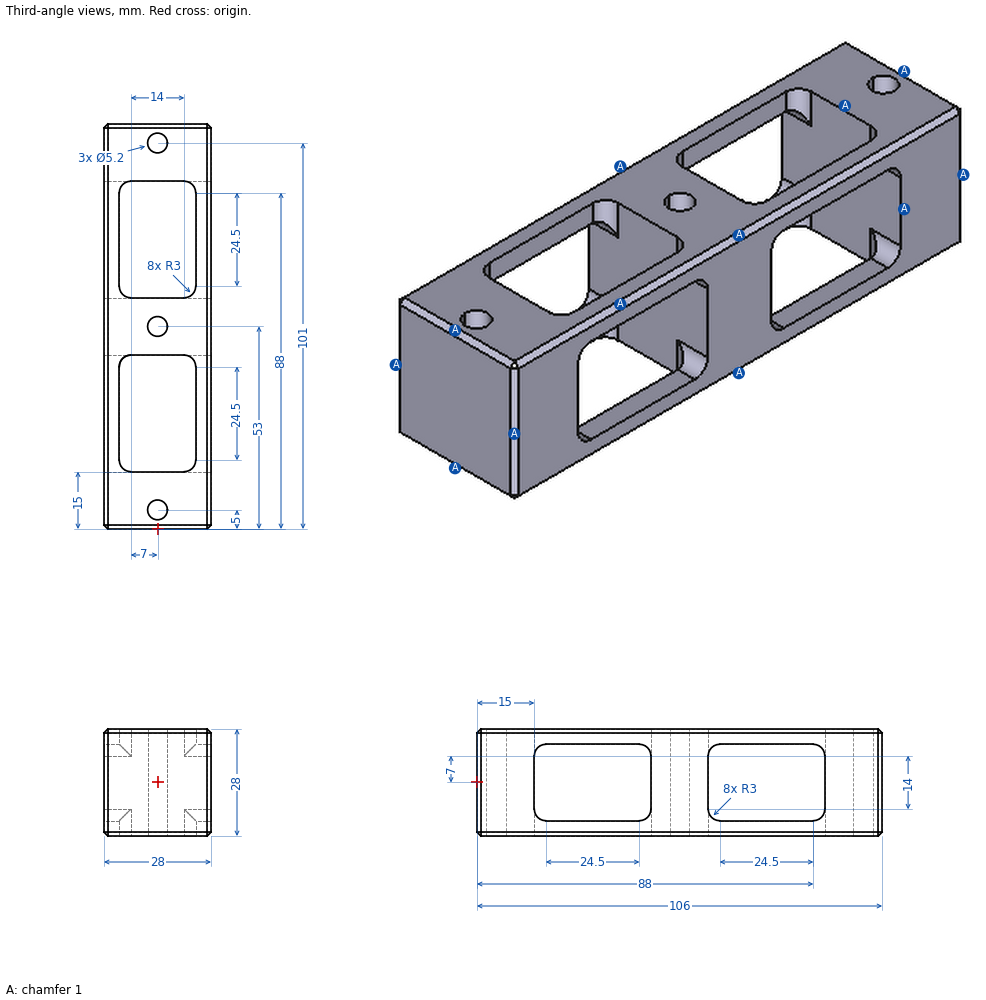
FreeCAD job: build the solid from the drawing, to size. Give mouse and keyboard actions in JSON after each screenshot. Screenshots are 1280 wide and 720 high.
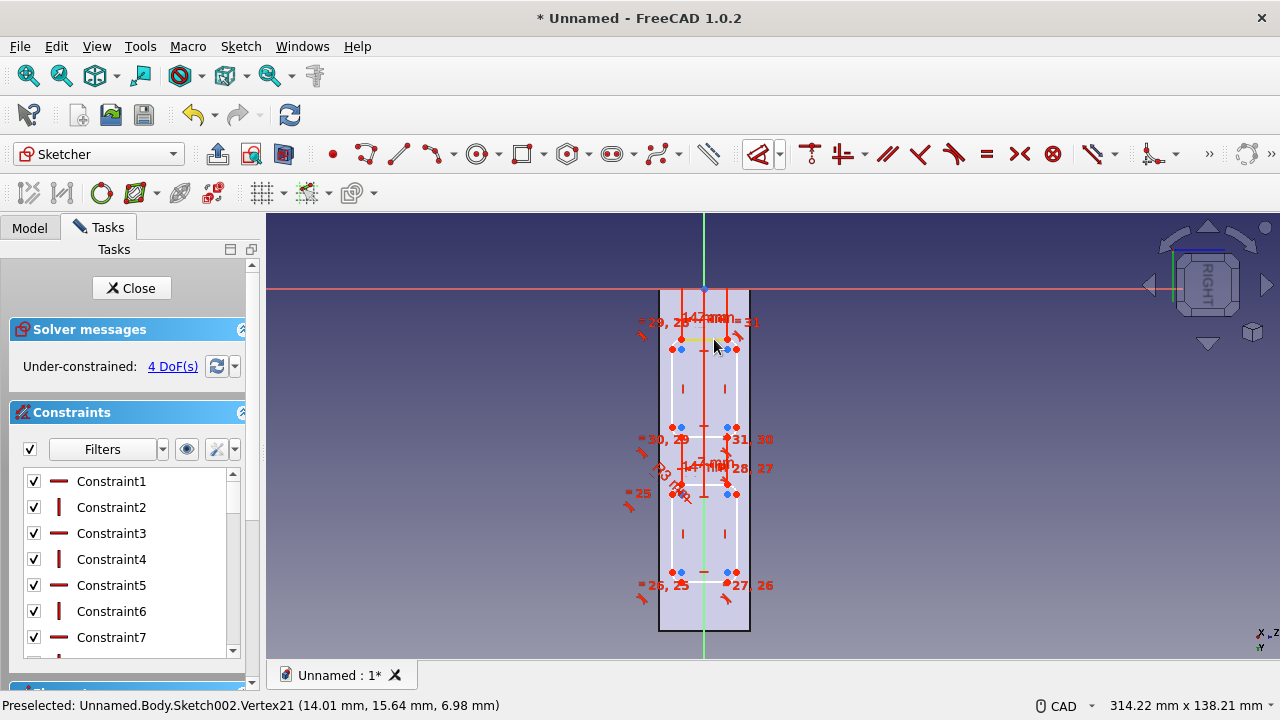
{"action": "scroll", "coordinate": [672, 573], "scroll_direction": "up", "scroll_amount": 2}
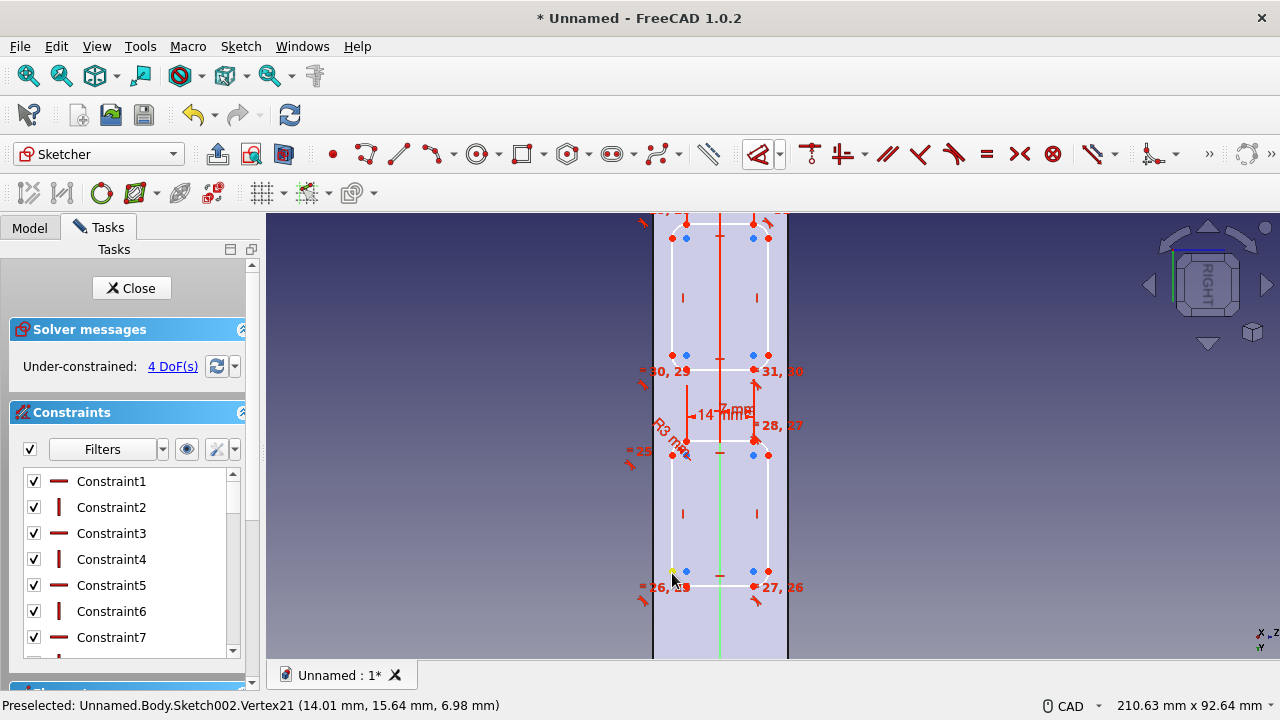
{"action": "left_click", "coordinate": [672, 572]}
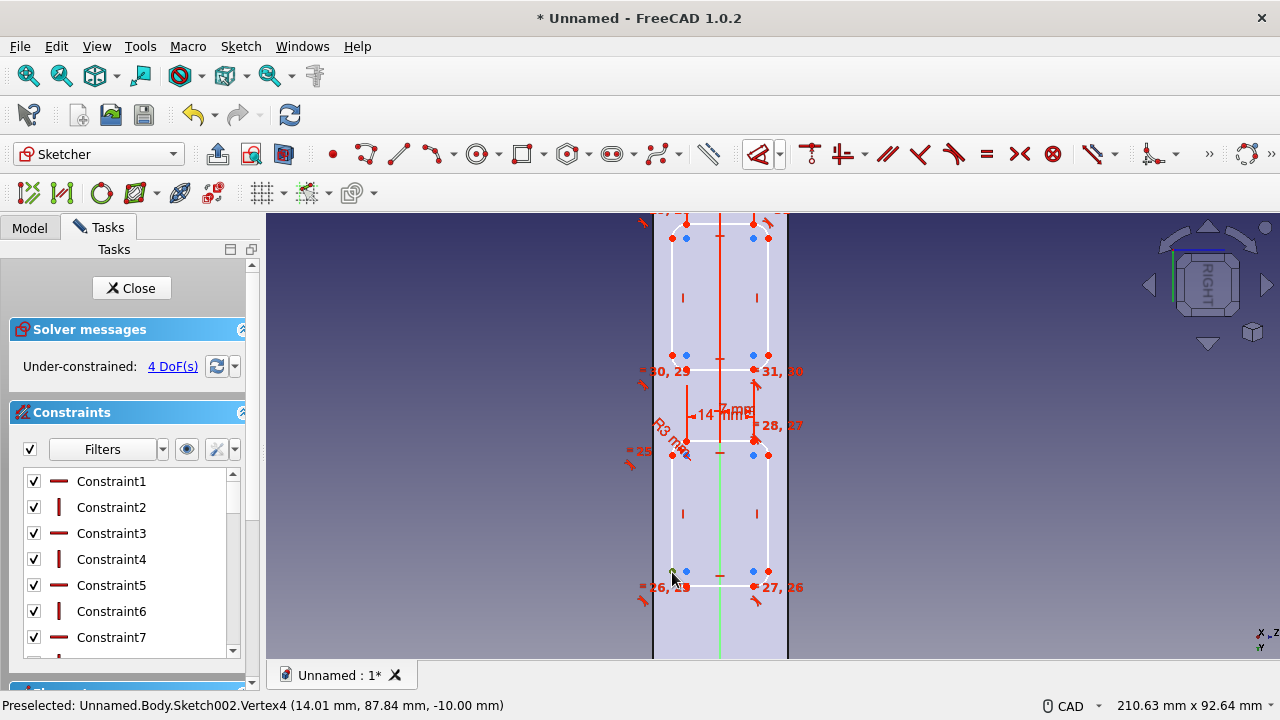
{"action": "key", "text": "i"}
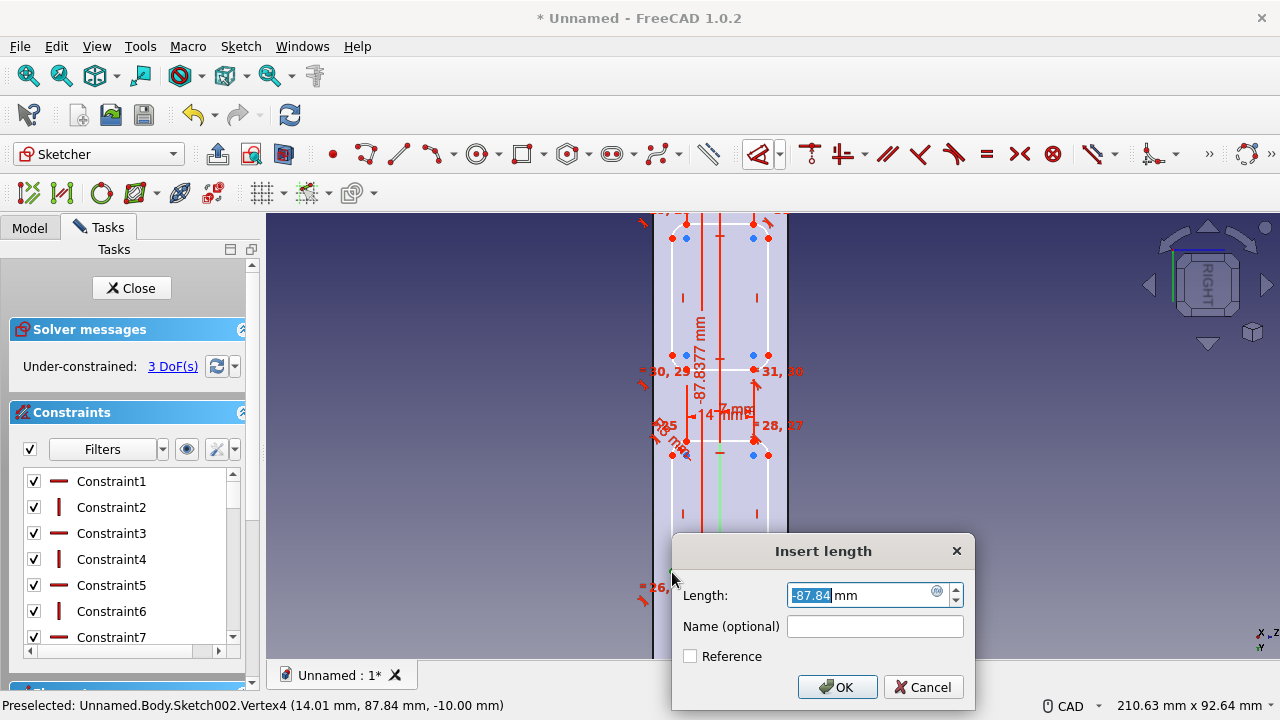
{"action": "type", "text": "-88"}
{"action": "key", "text": "Return"}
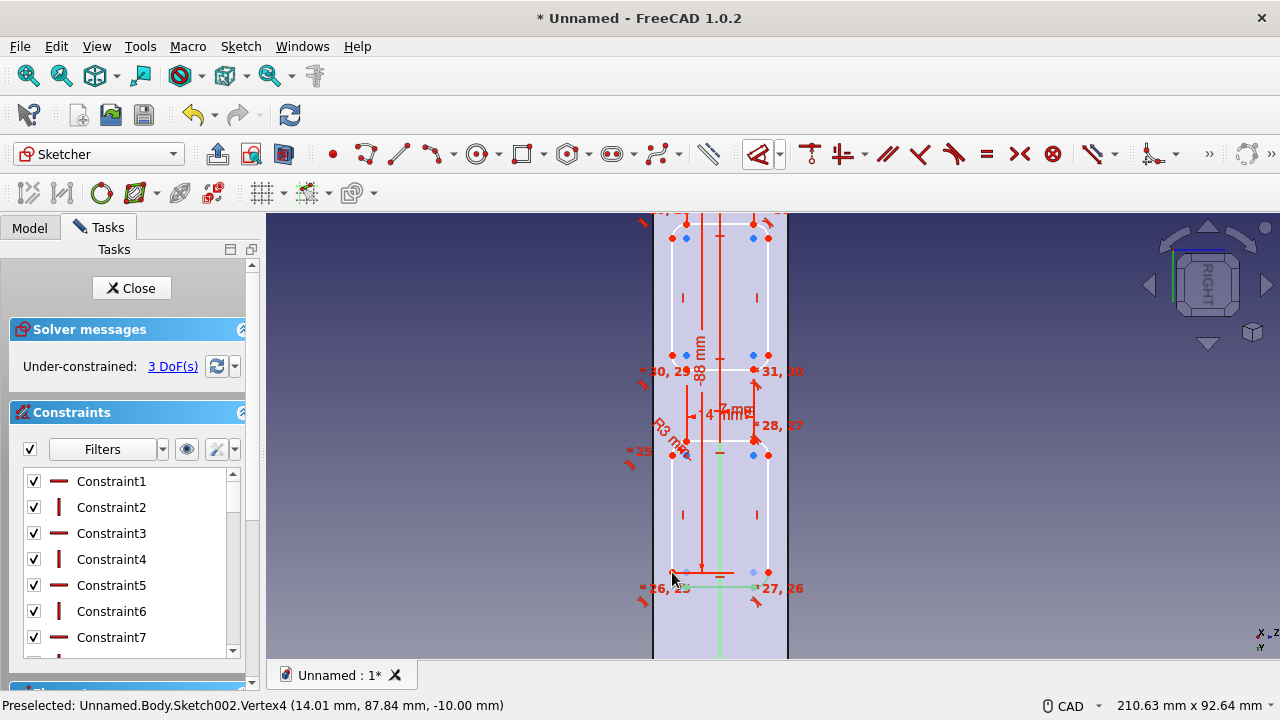
{"action": "scroll", "coordinate": [672, 574], "scroll_direction": "down", "scroll_amount": 2}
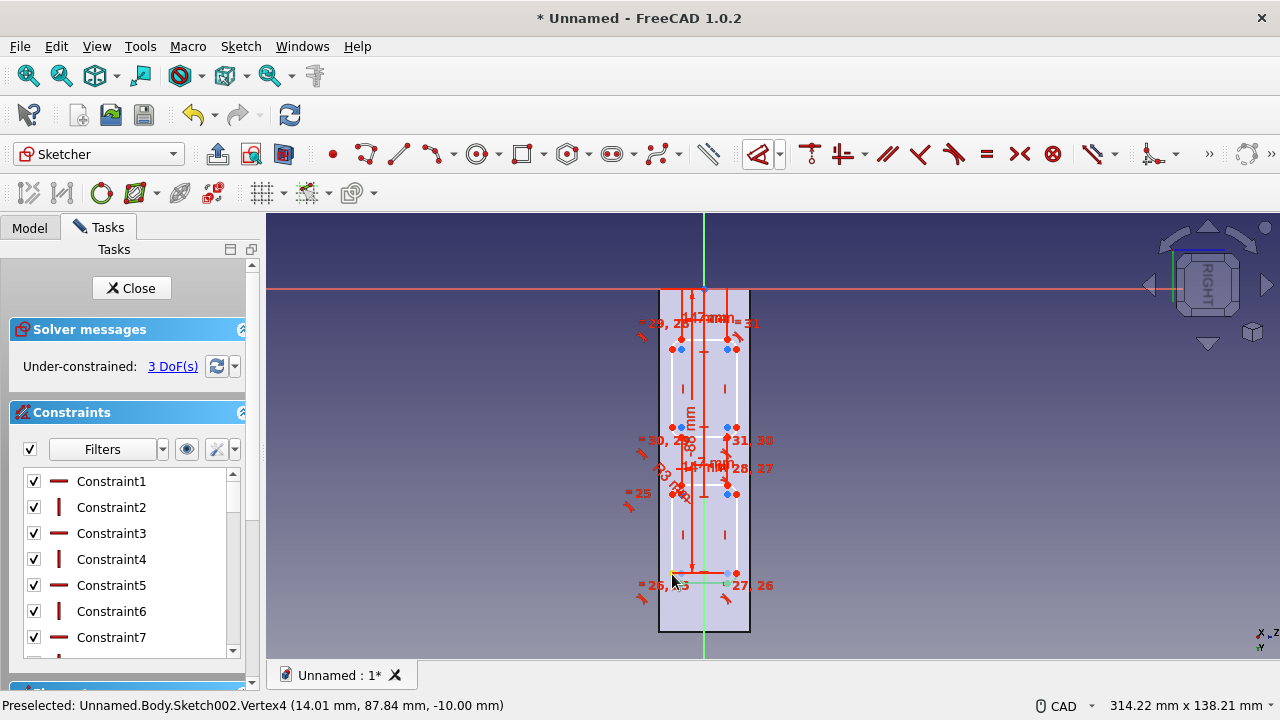
{"action": "scroll", "coordinate": [727, 340], "scroll_direction": "up", "scroll_amount": 2}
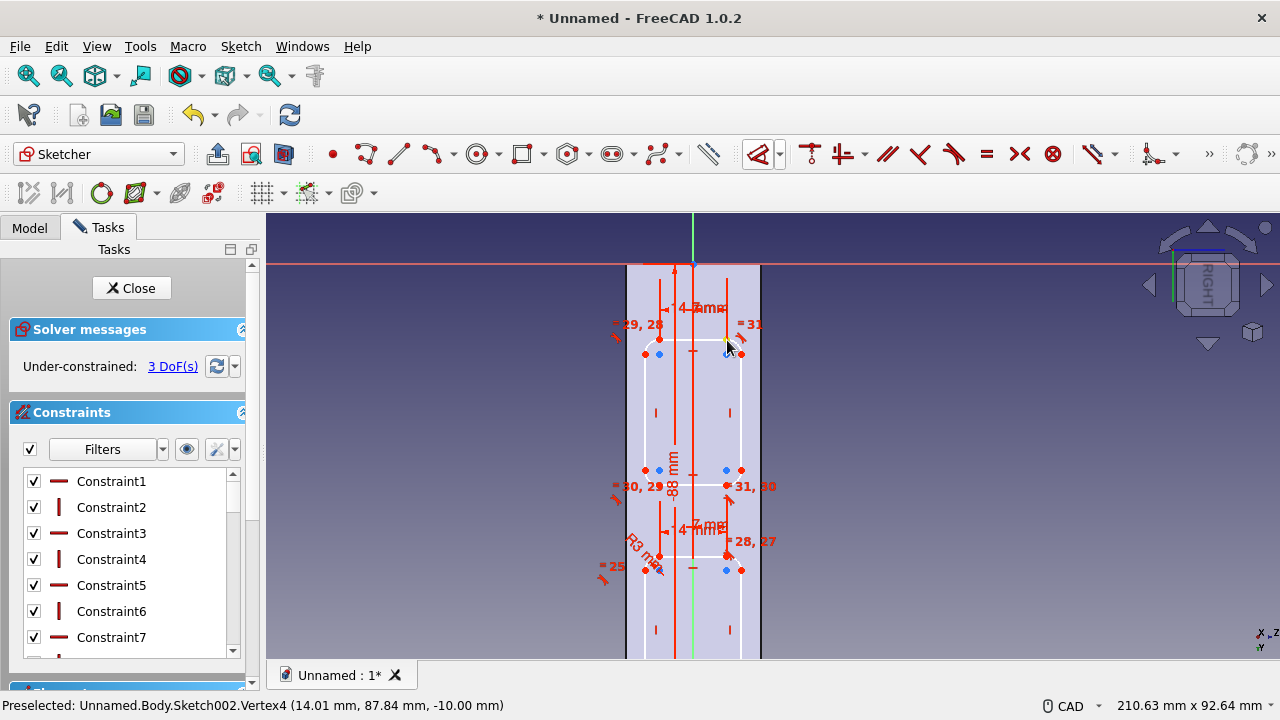
{"action": "left_click", "coordinate": [727, 340]}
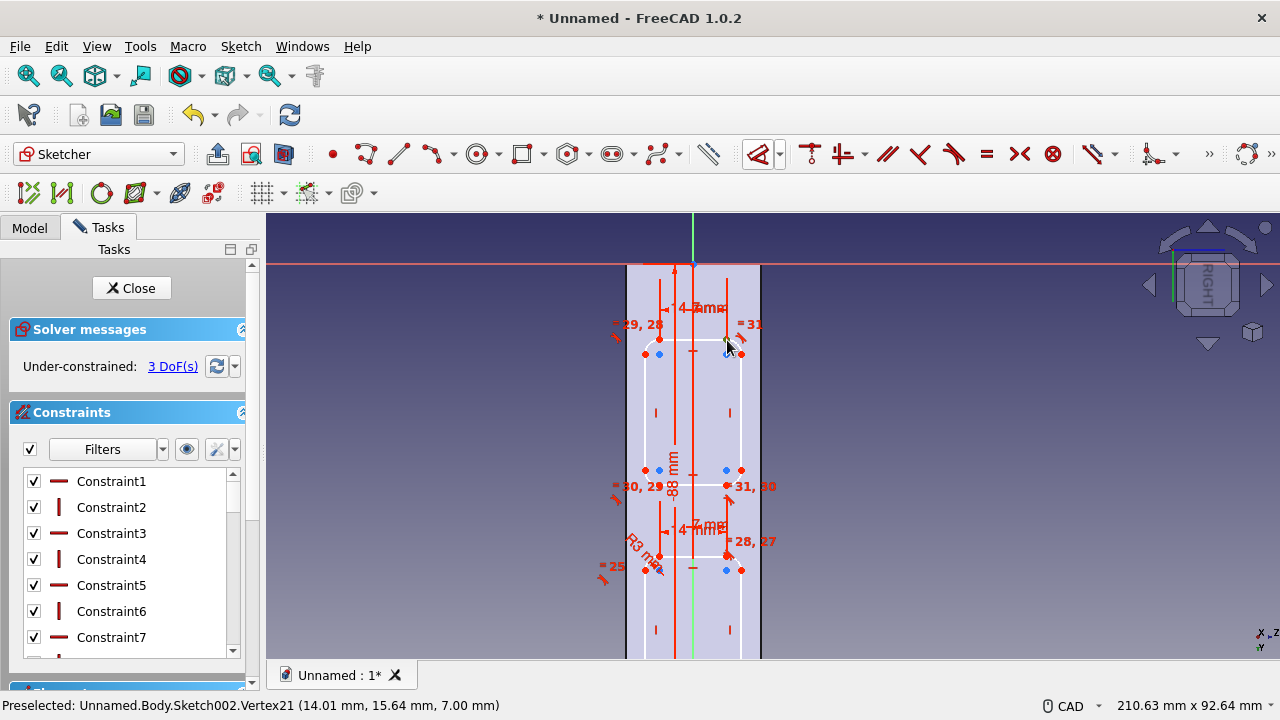
{"action": "key", "text": "i"}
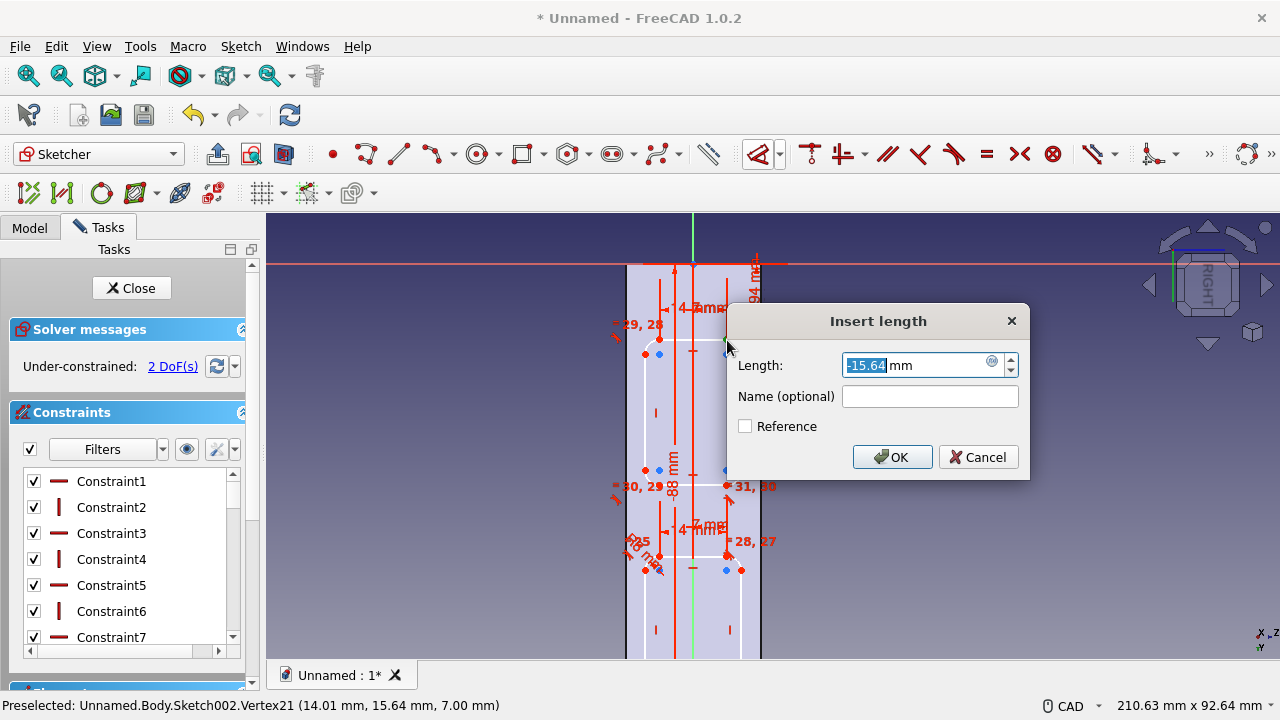
{"action": "type", "text": "-15"}
{"action": "key", "text": "Return"}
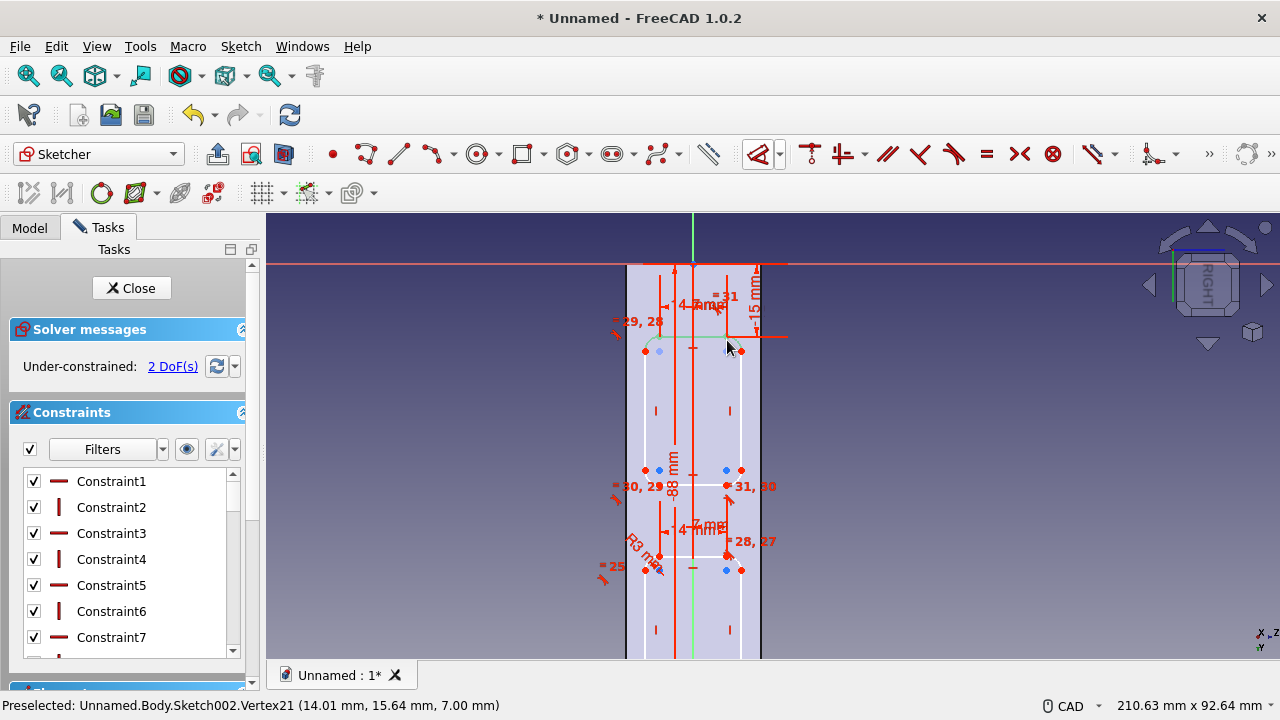
{"action": "left_click", "coordinate": [645, 606]}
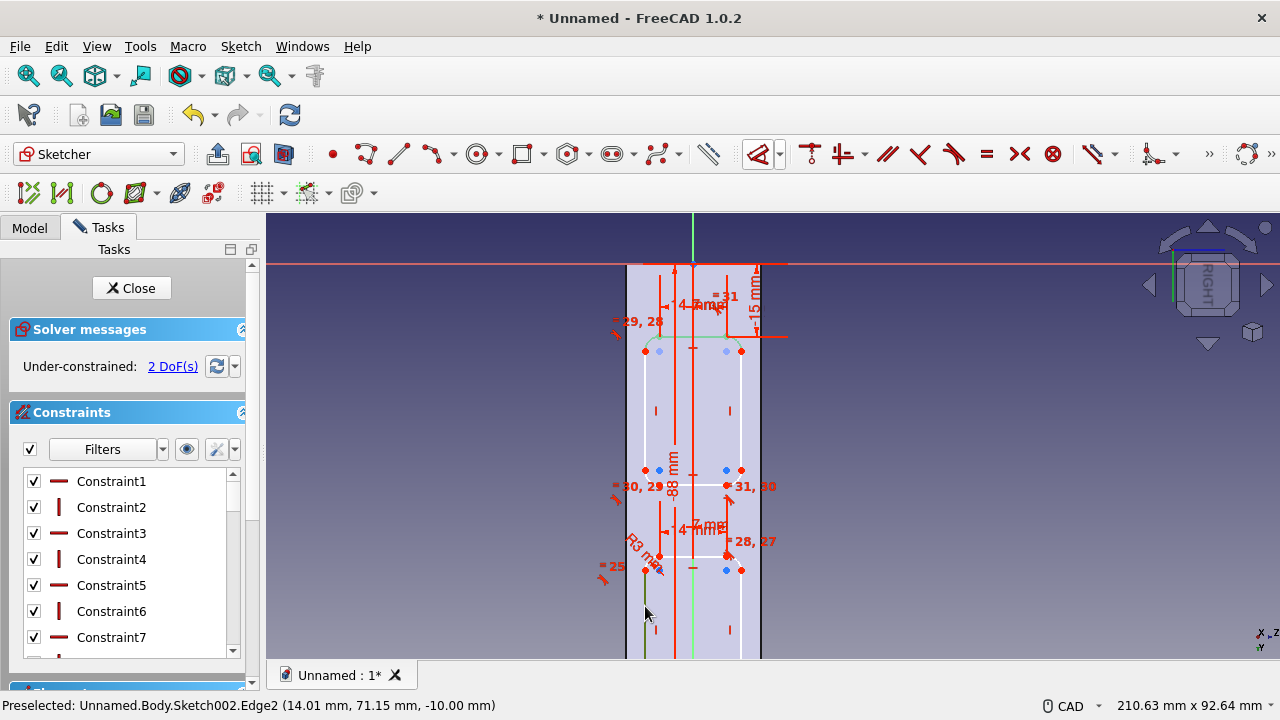
{"action": "left_click", "coordinate": [780, 154]}